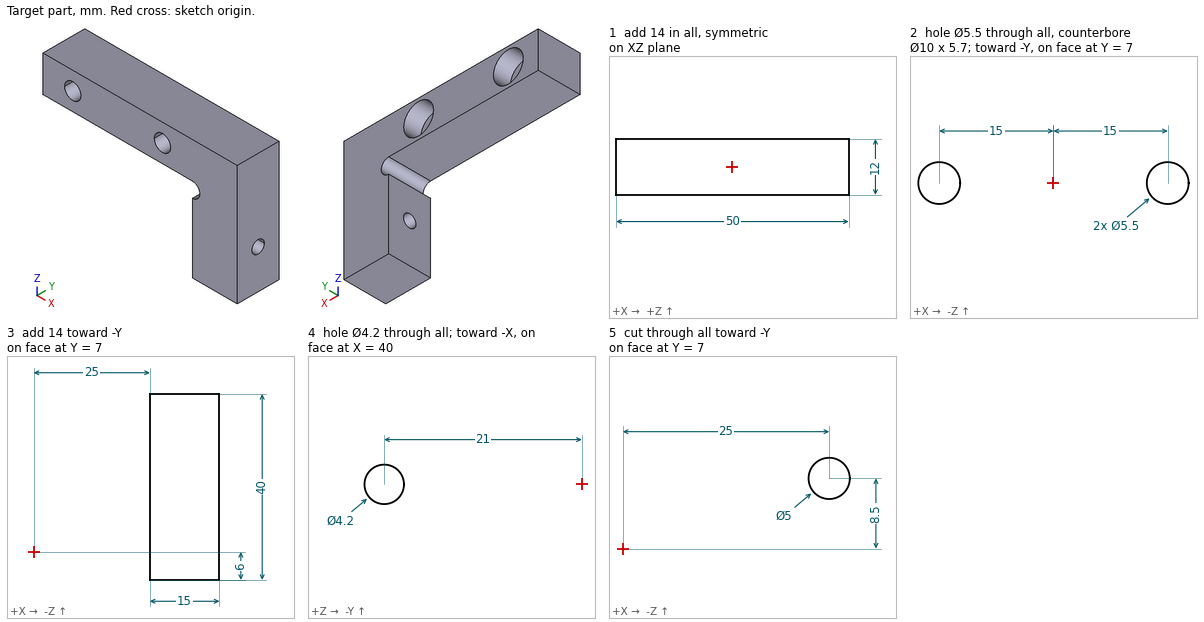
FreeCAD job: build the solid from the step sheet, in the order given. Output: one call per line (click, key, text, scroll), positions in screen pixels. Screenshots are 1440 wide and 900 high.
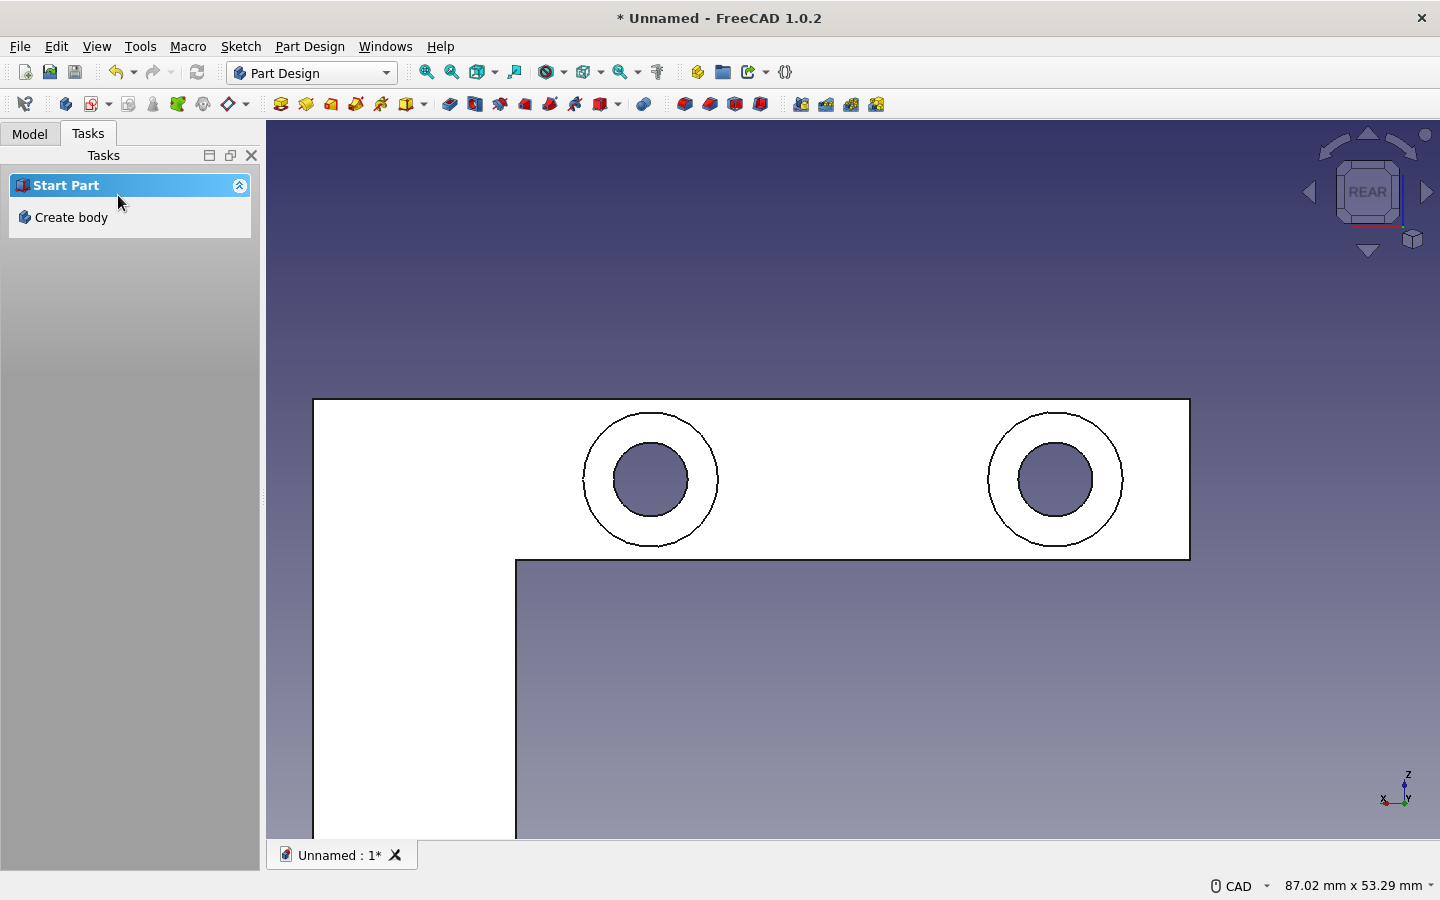
click(427, 72)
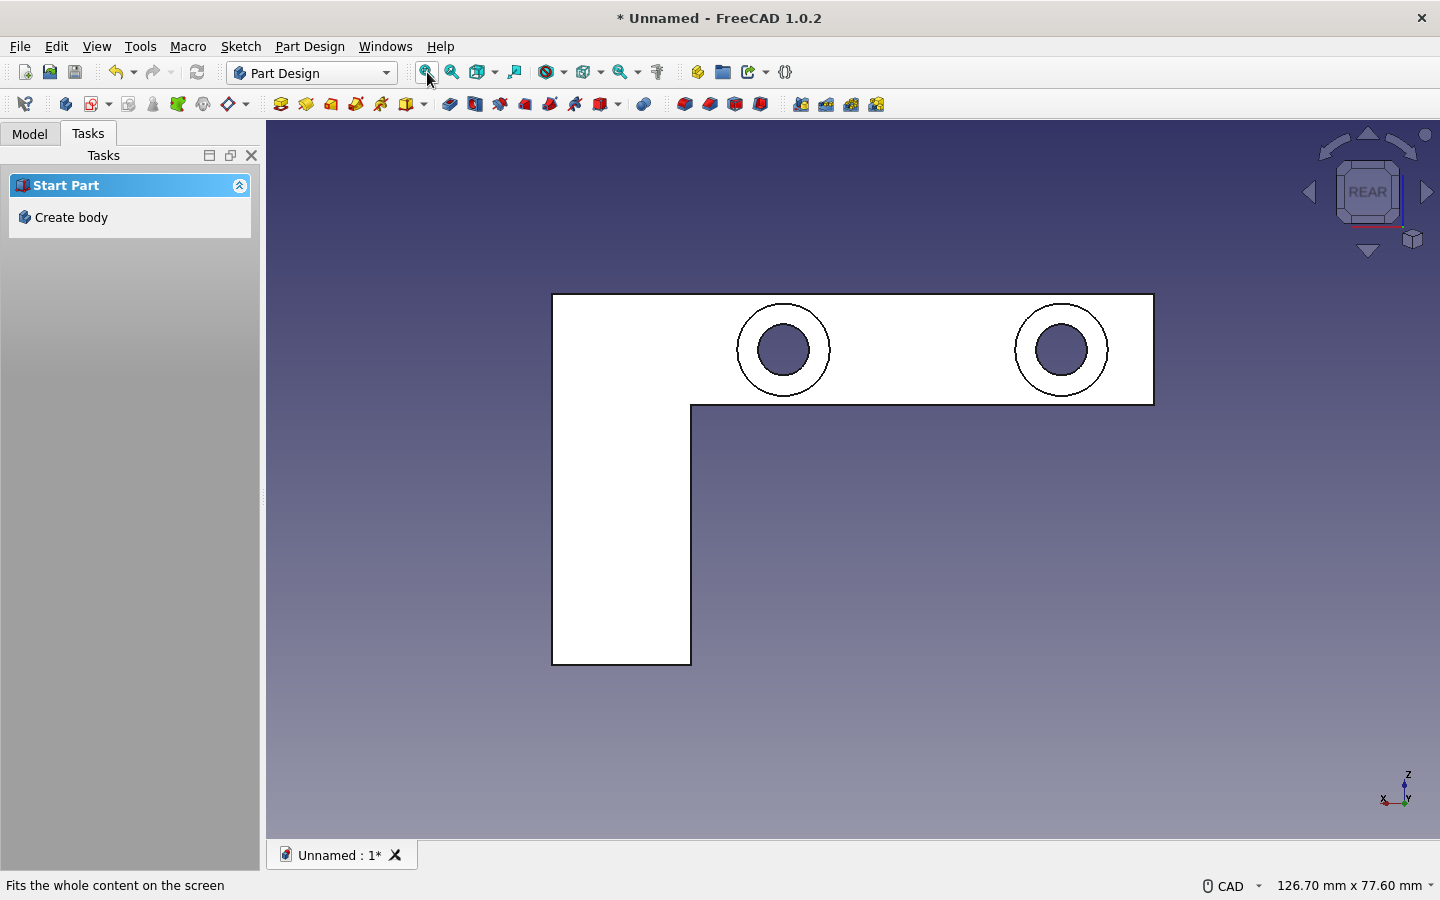
key(0)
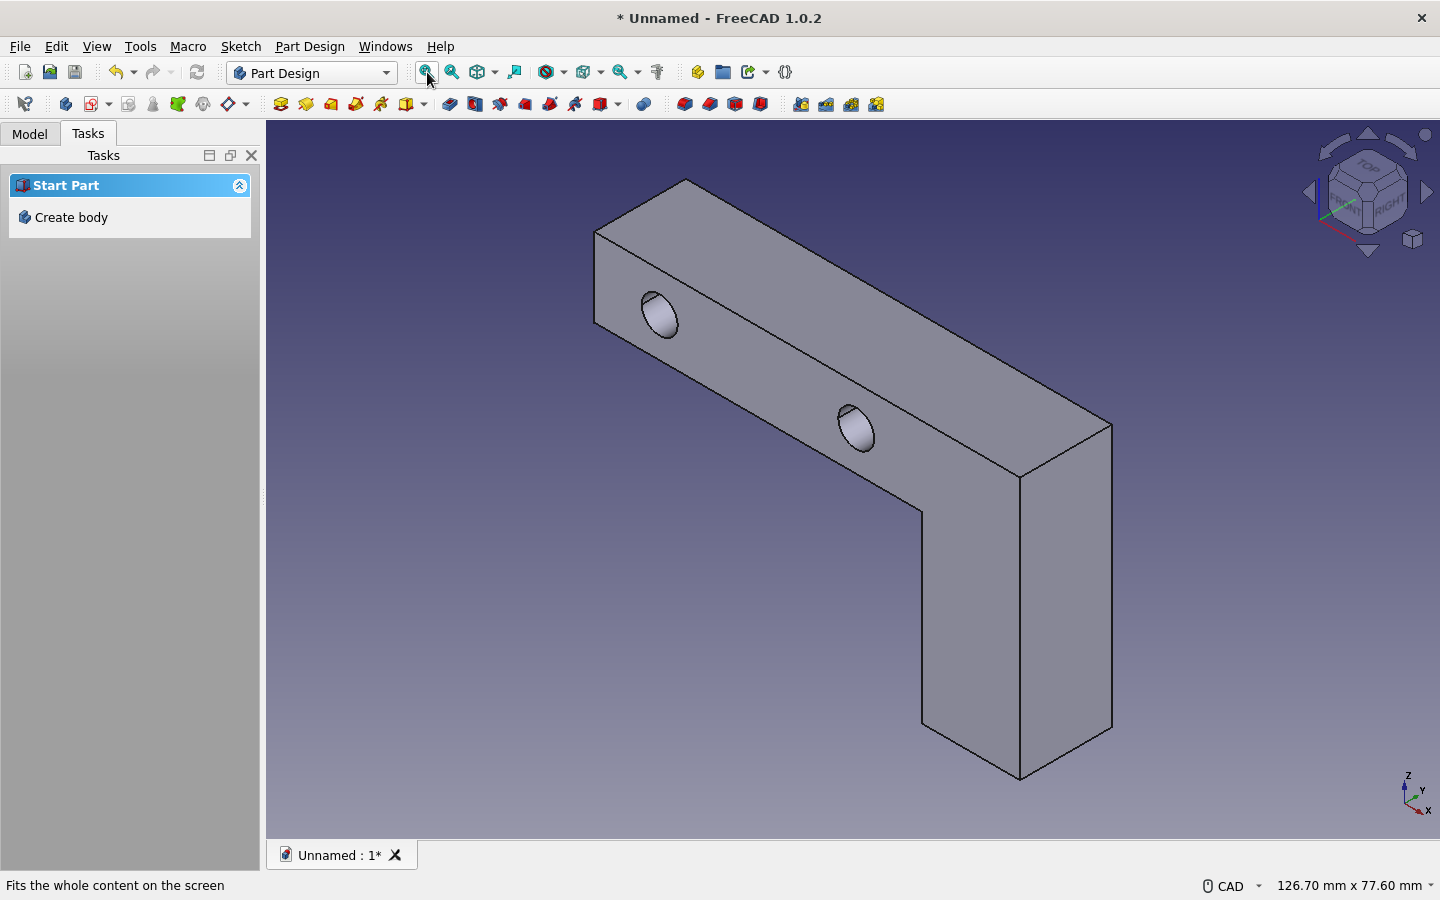
click(1066, 645)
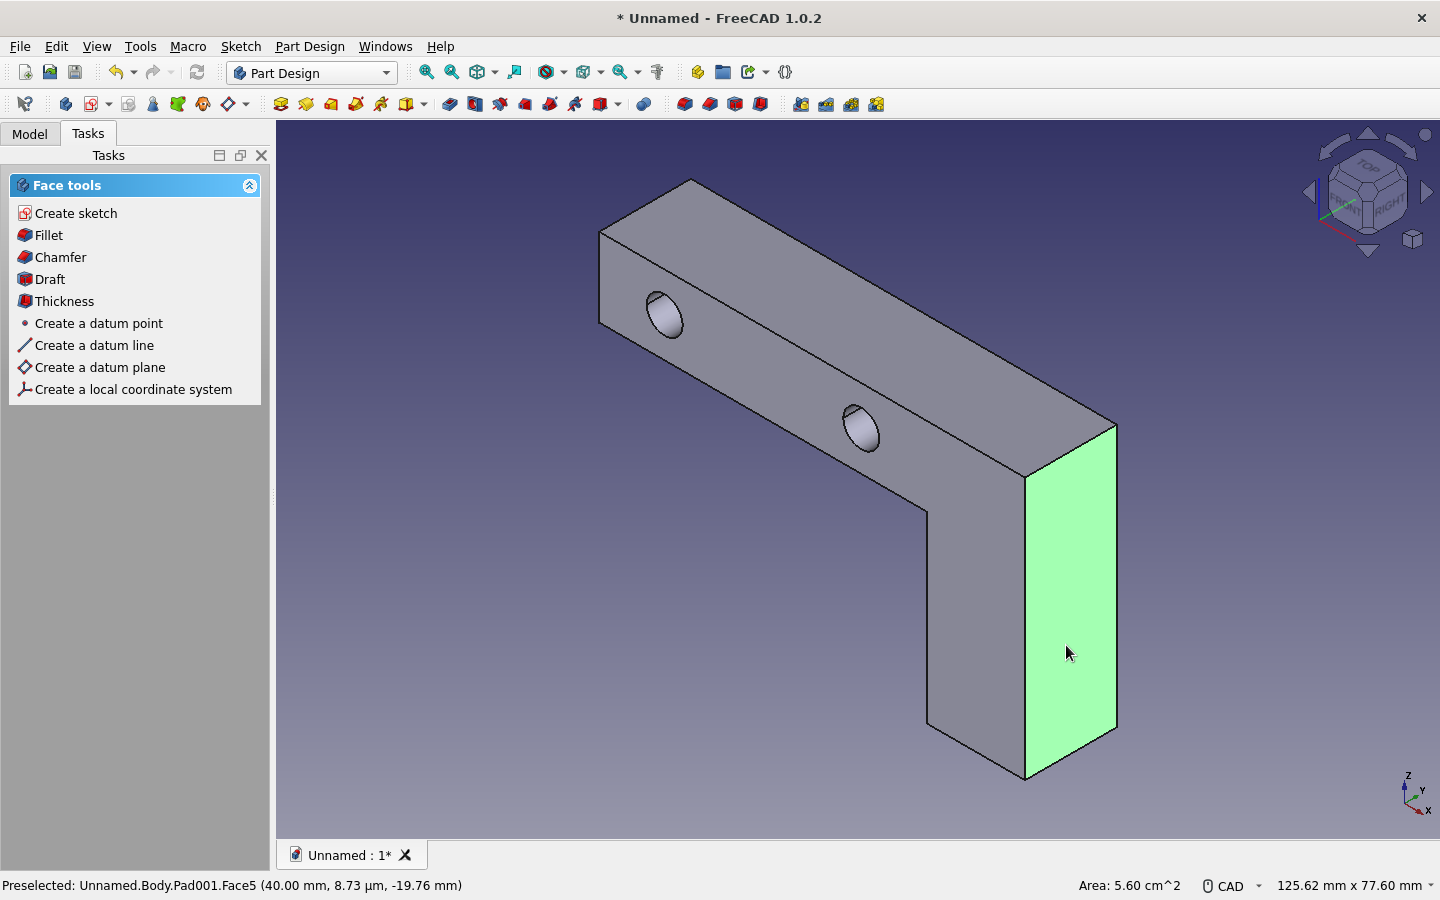
click(90, 104)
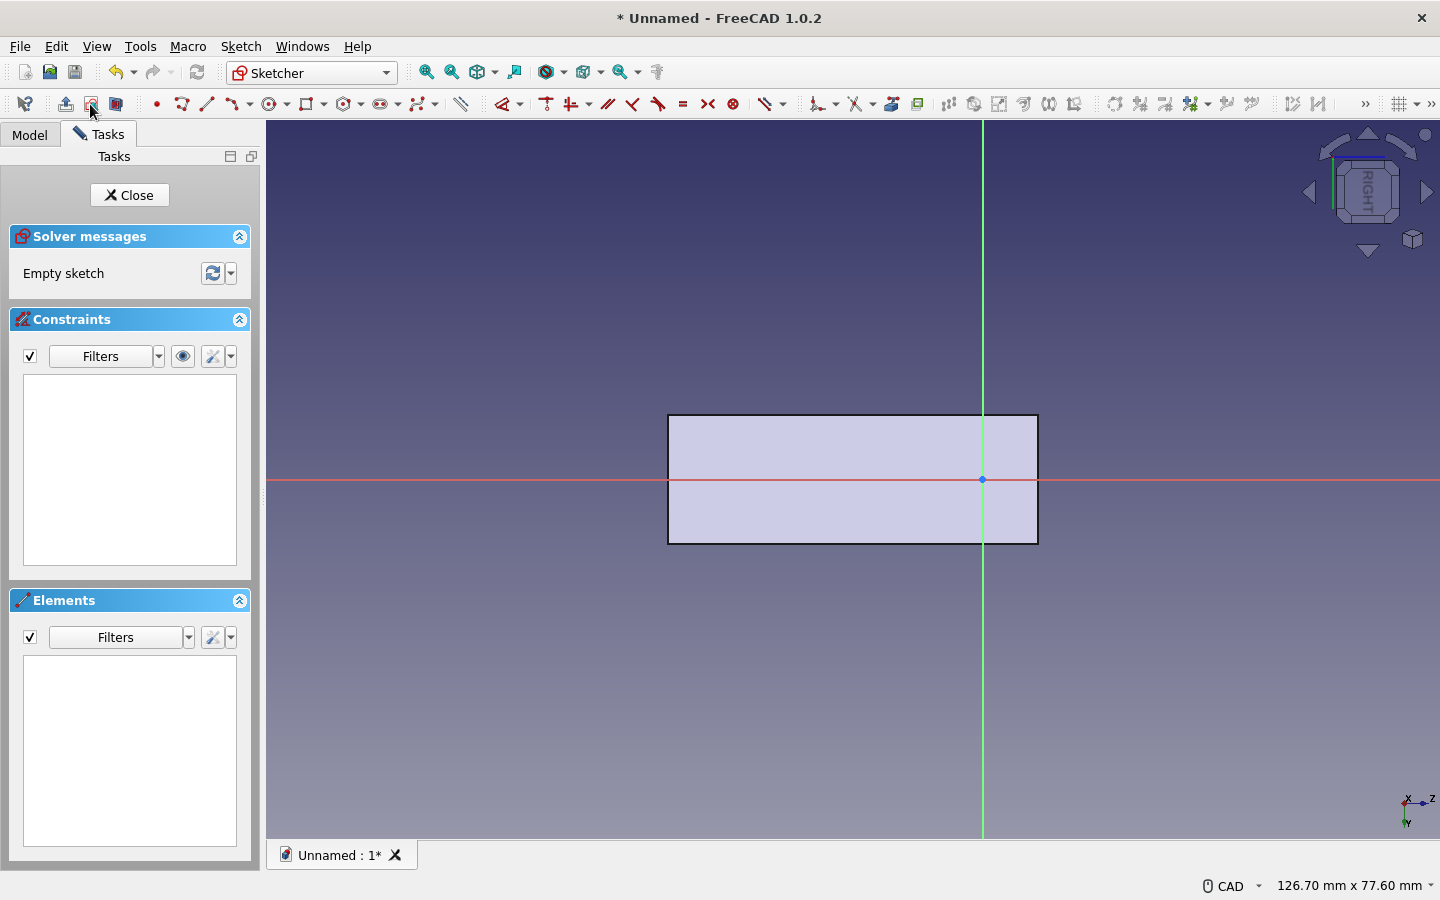
scroll(789, 480, up, 12)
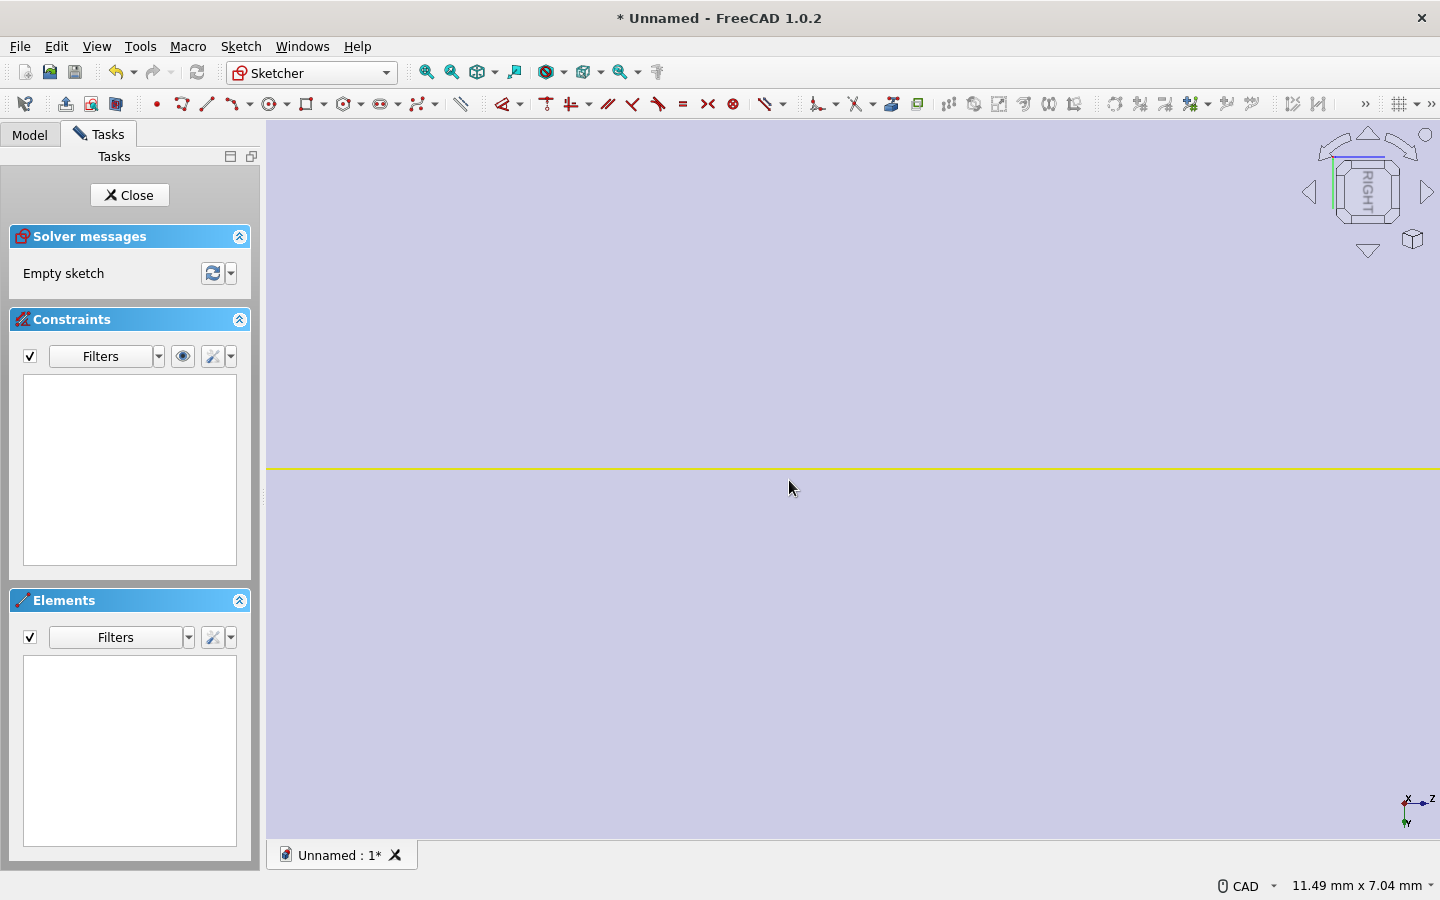
click(268, 104)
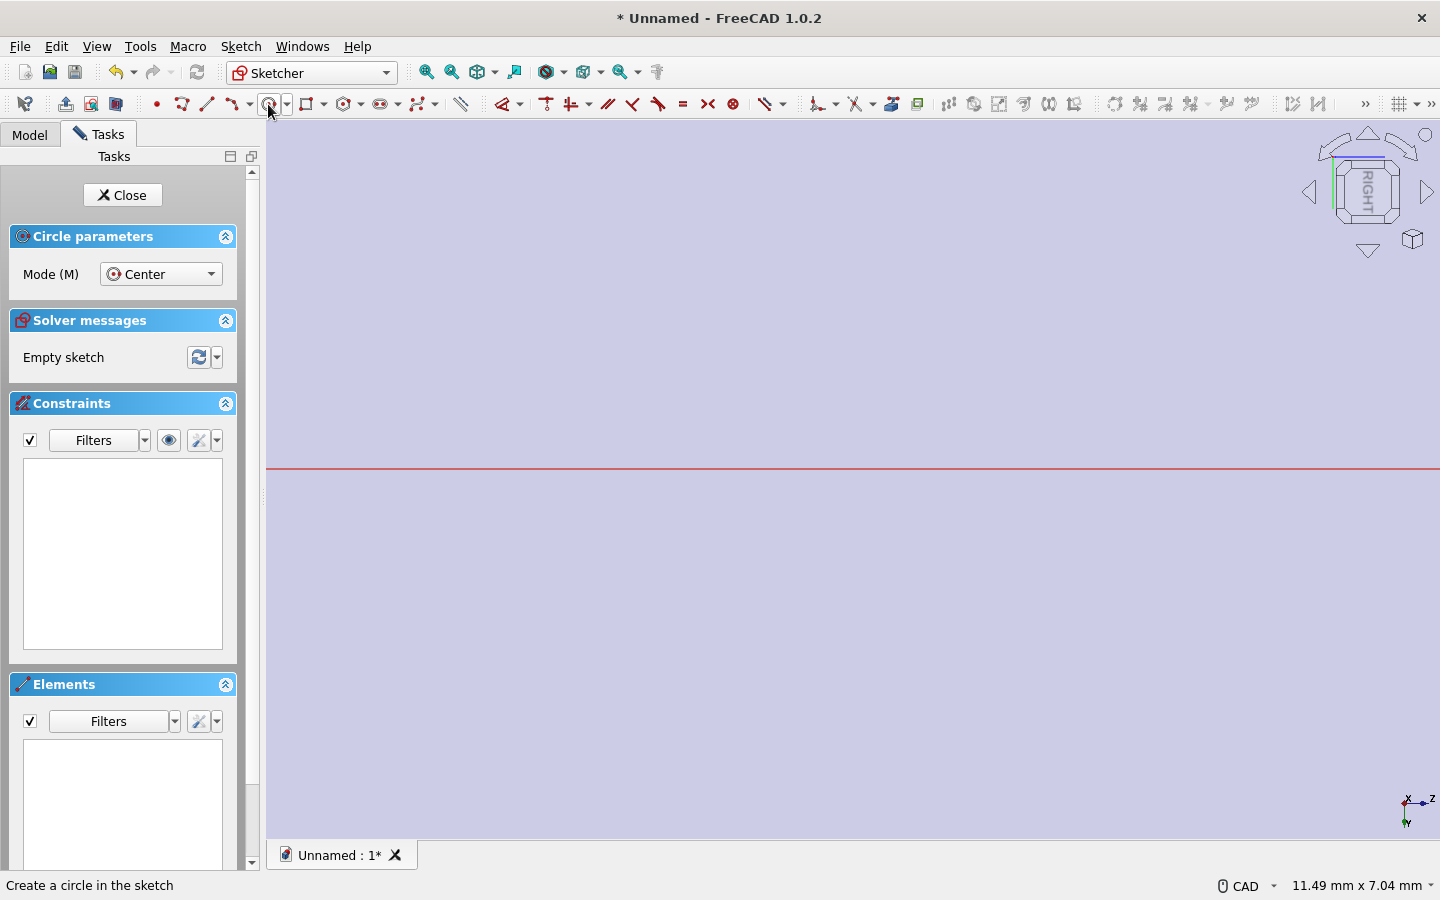
click(775, 469)
move(927, 318)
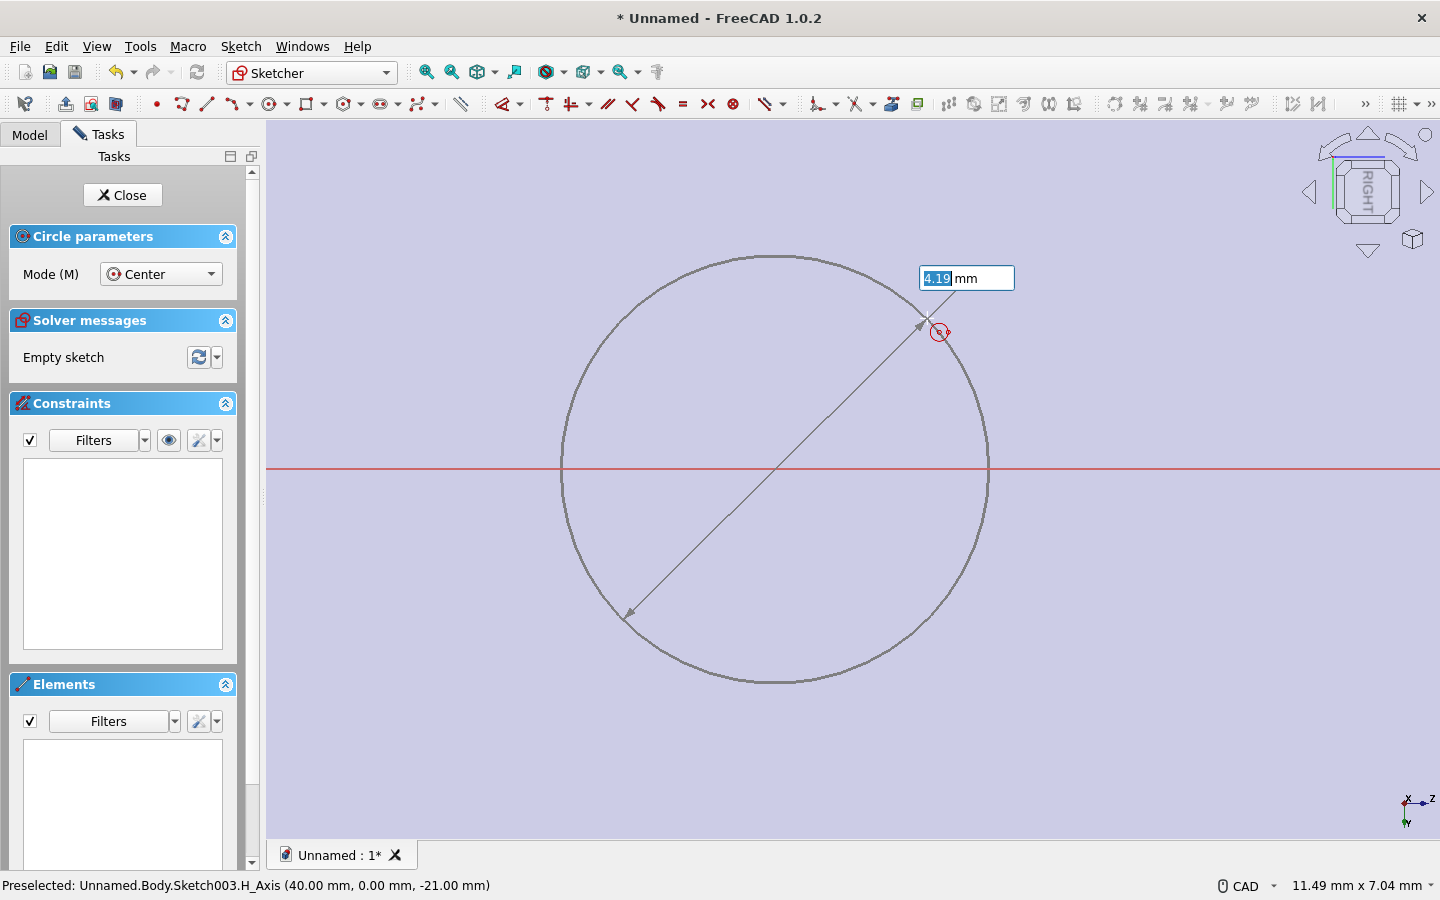
text(4.2)
key(Return)
key(Escape)